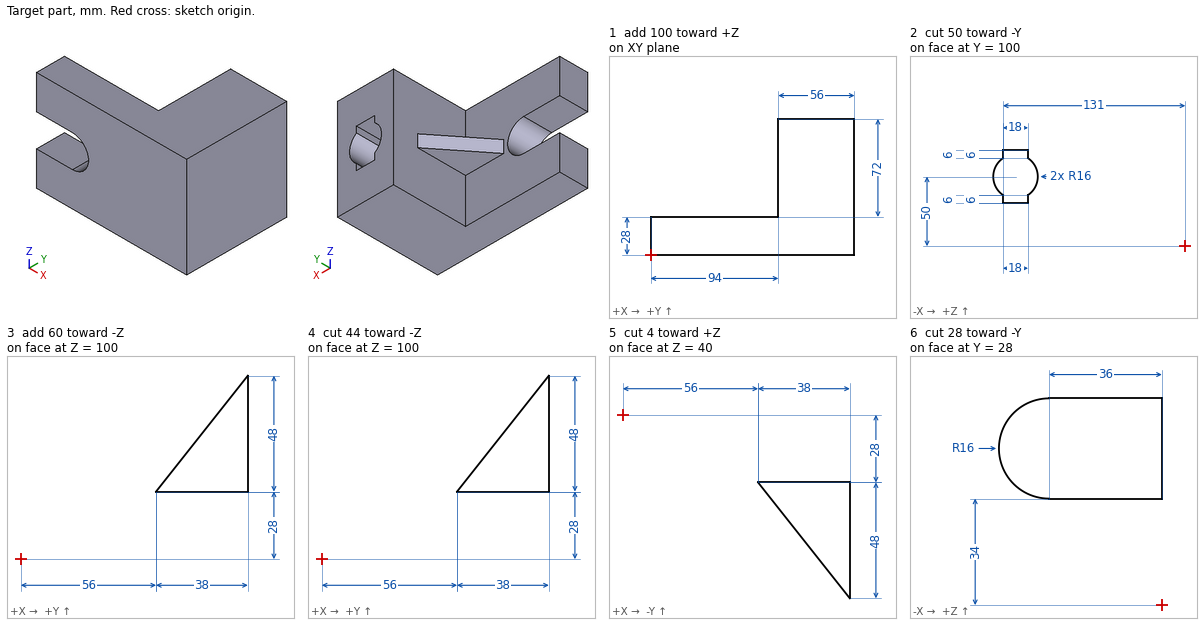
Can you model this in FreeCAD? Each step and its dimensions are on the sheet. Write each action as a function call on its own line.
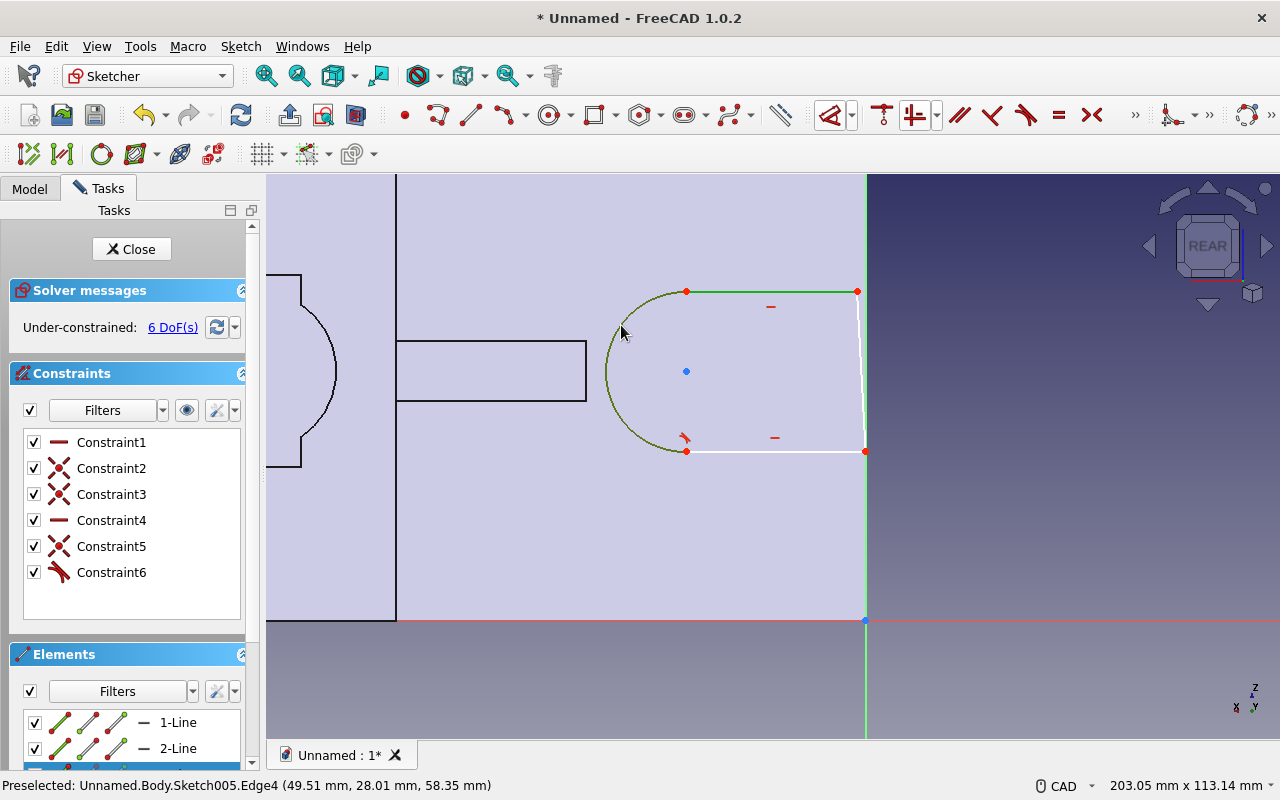
click(1026, 116)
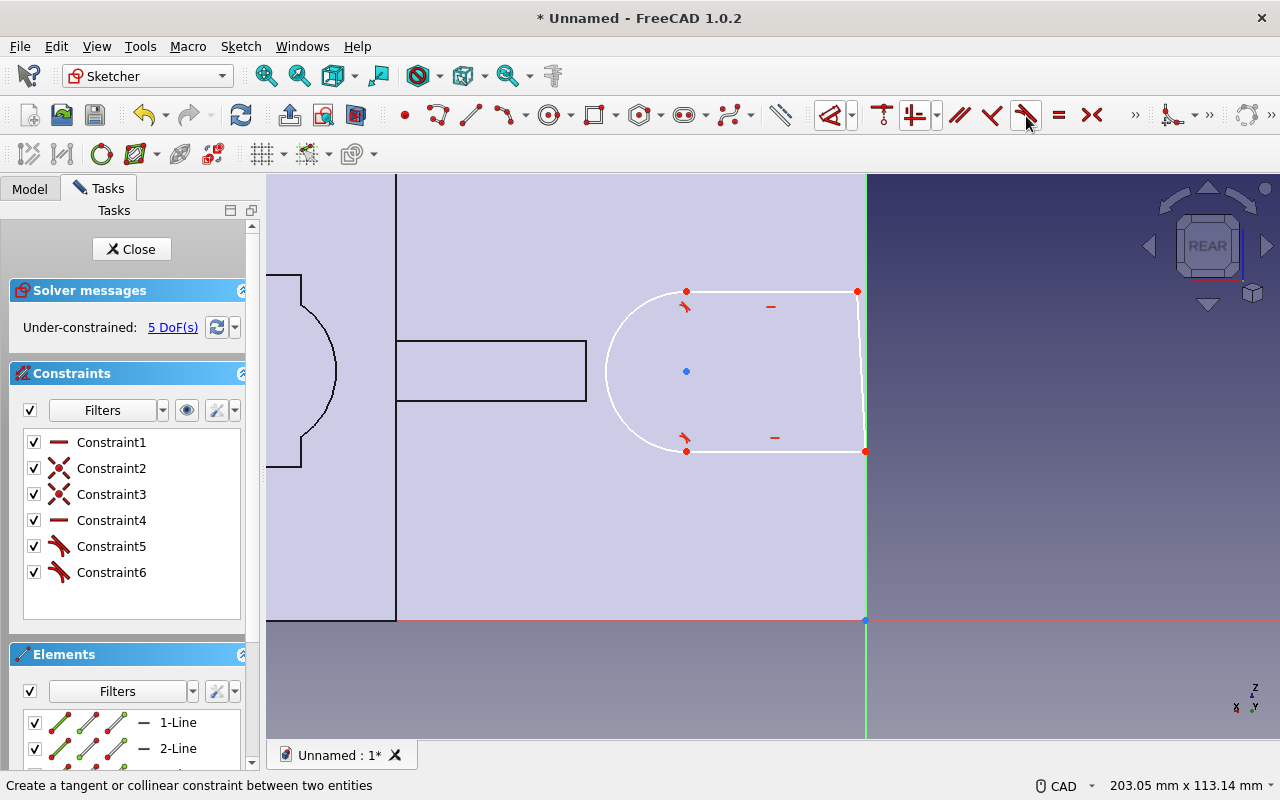
click(863, 404)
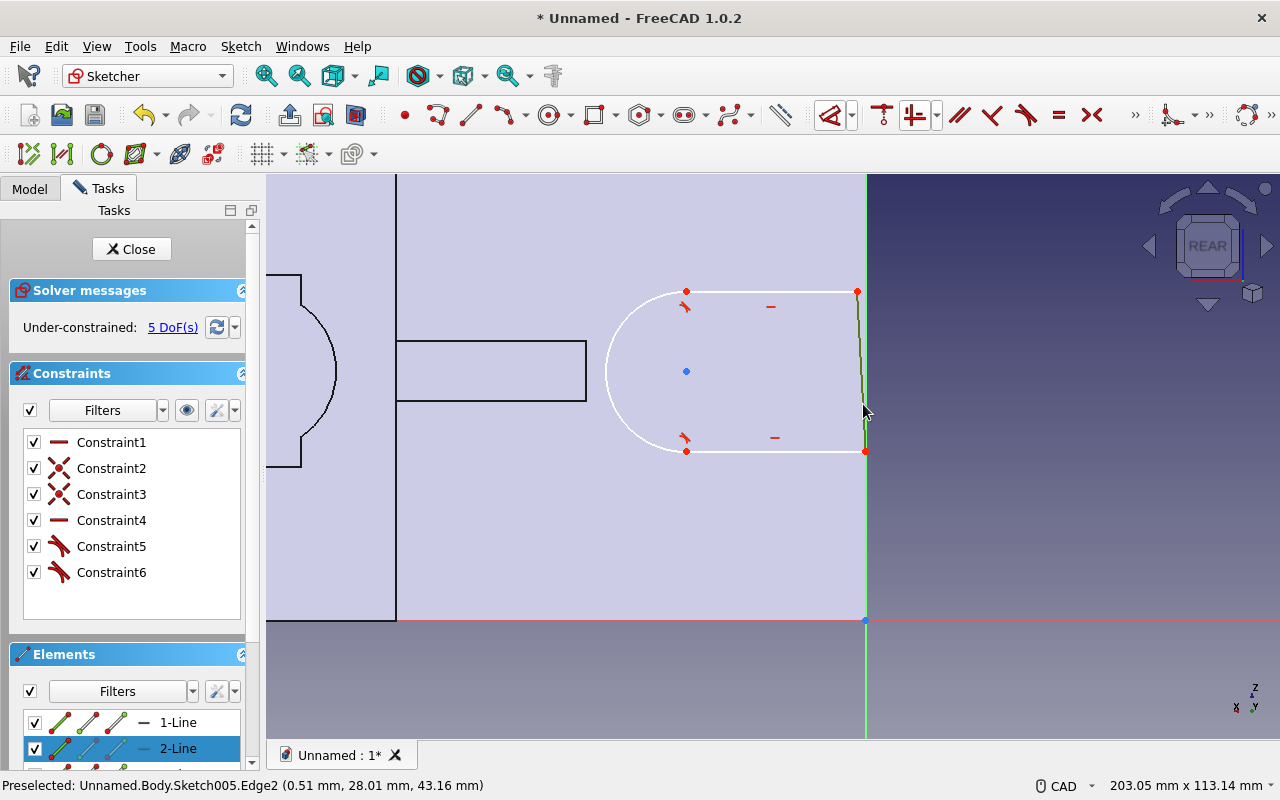
key(v)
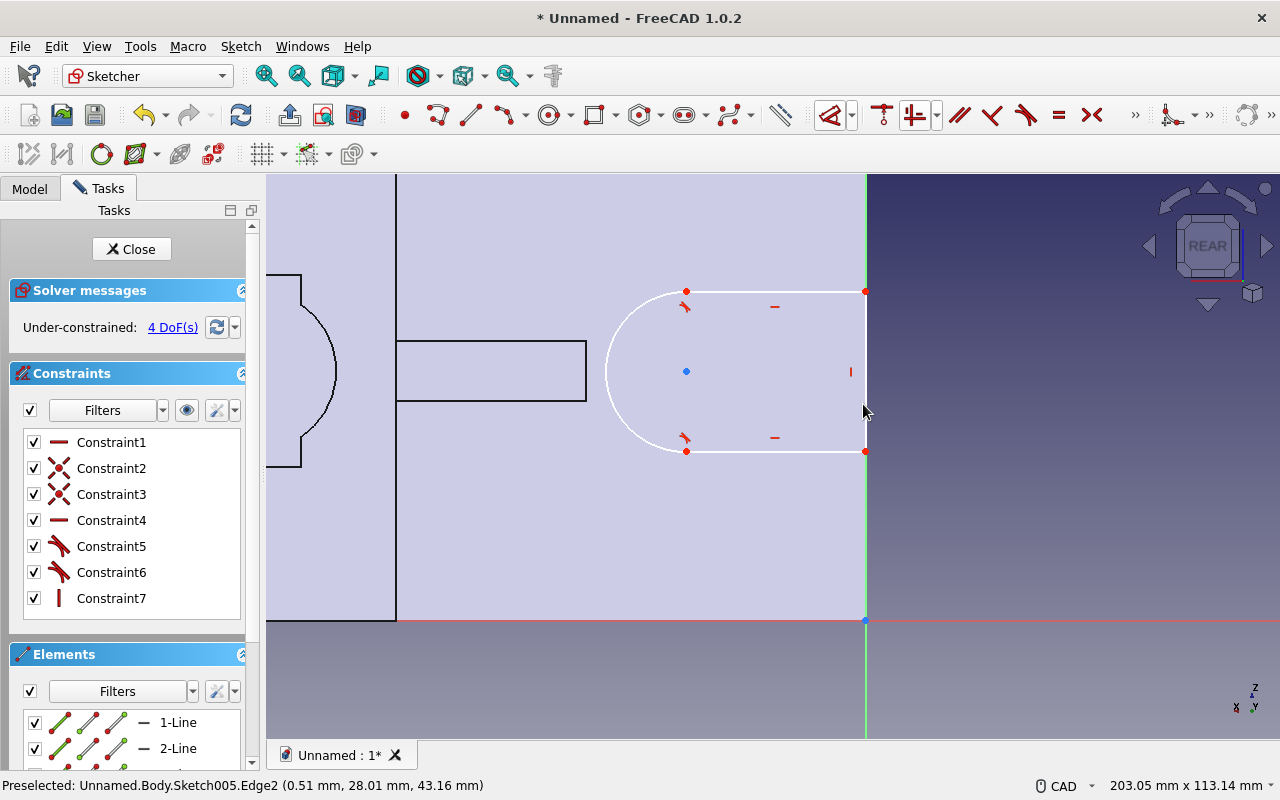
click(621, 325)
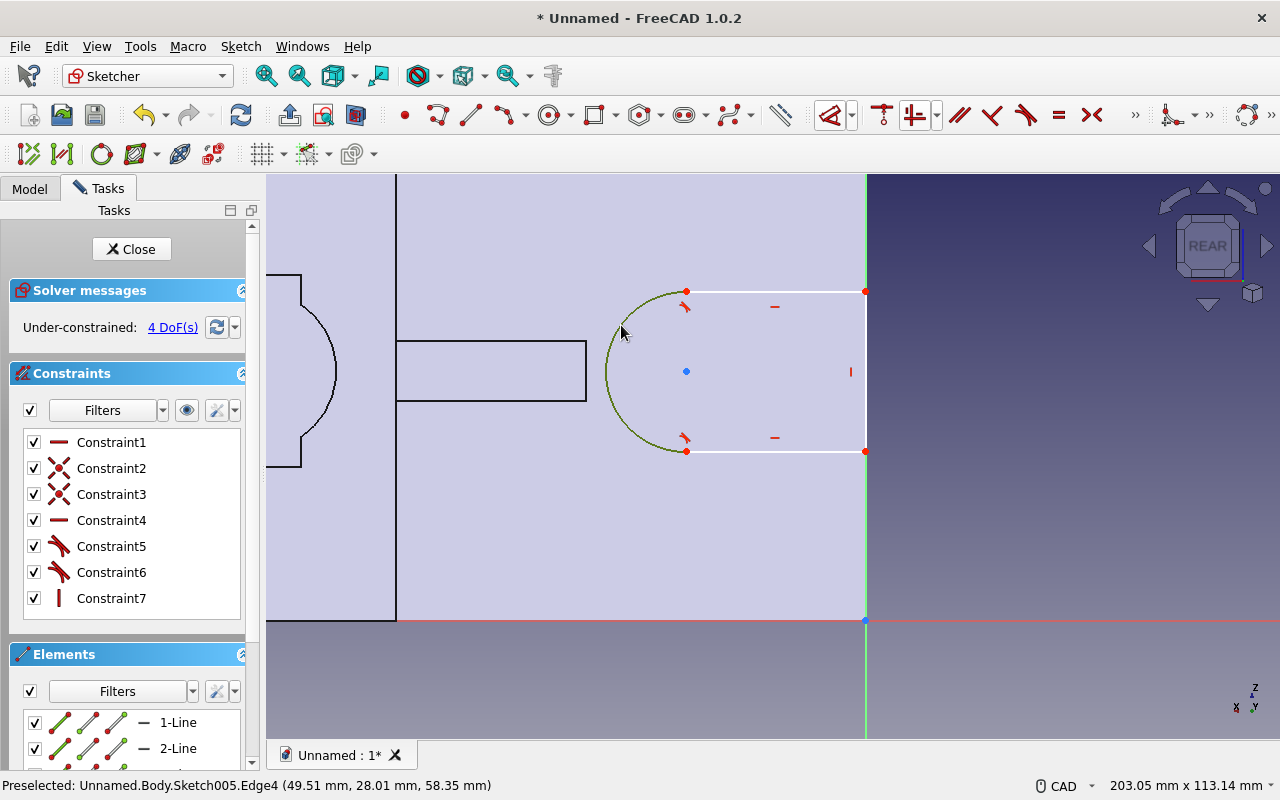
click(852, 116)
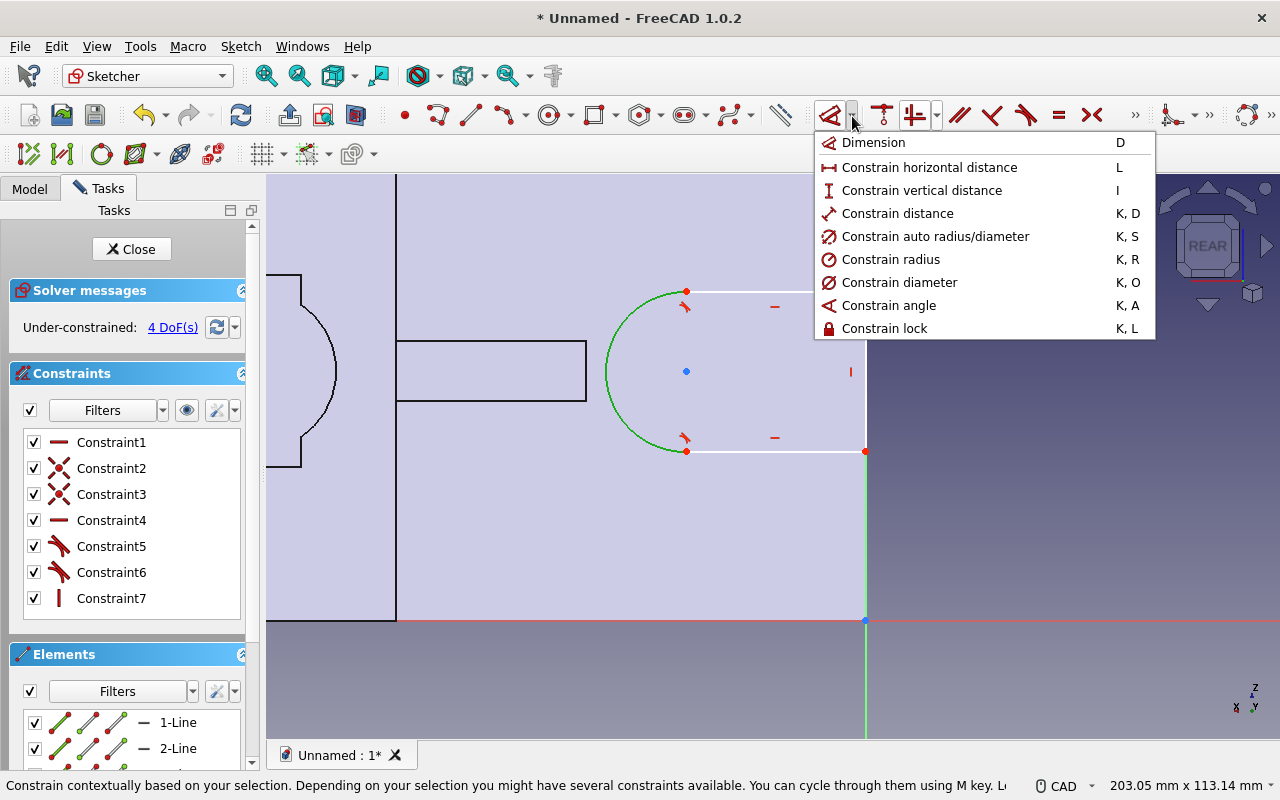
click(985, 260)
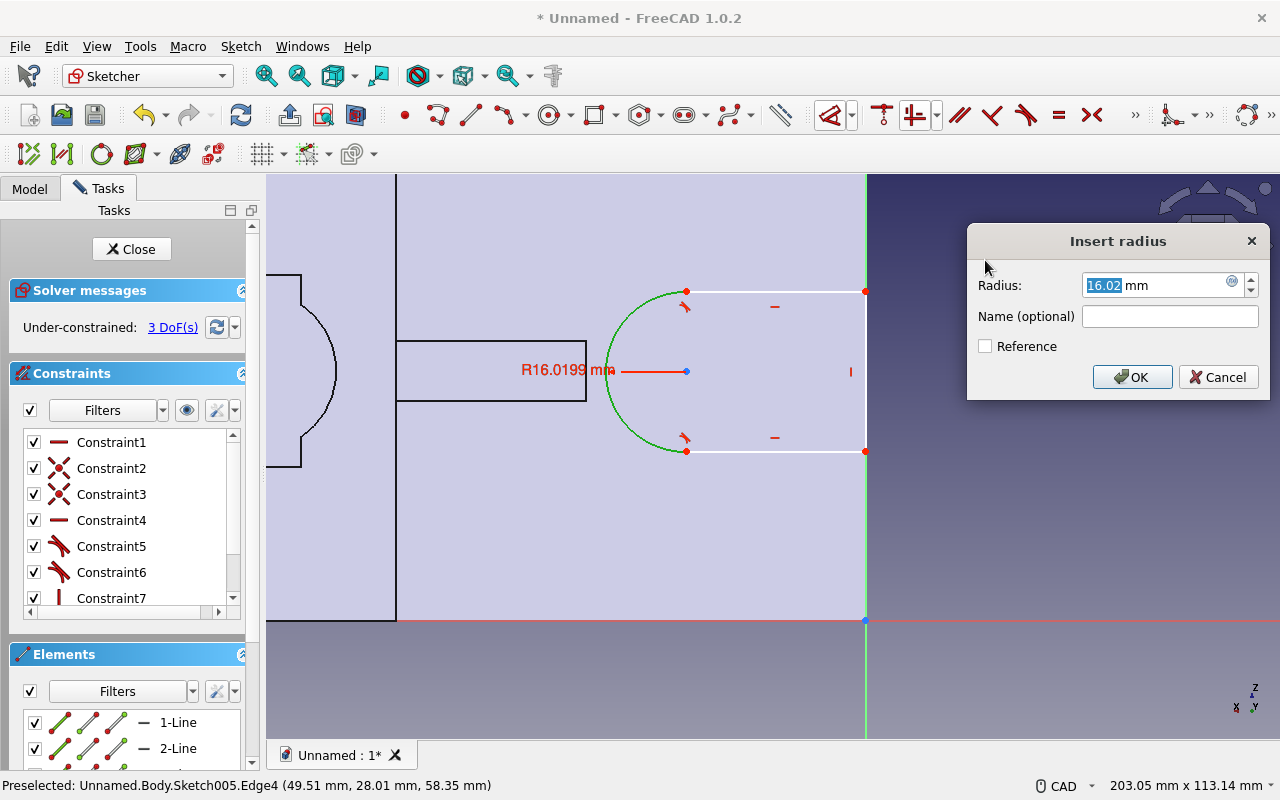
text(16)
key(Return)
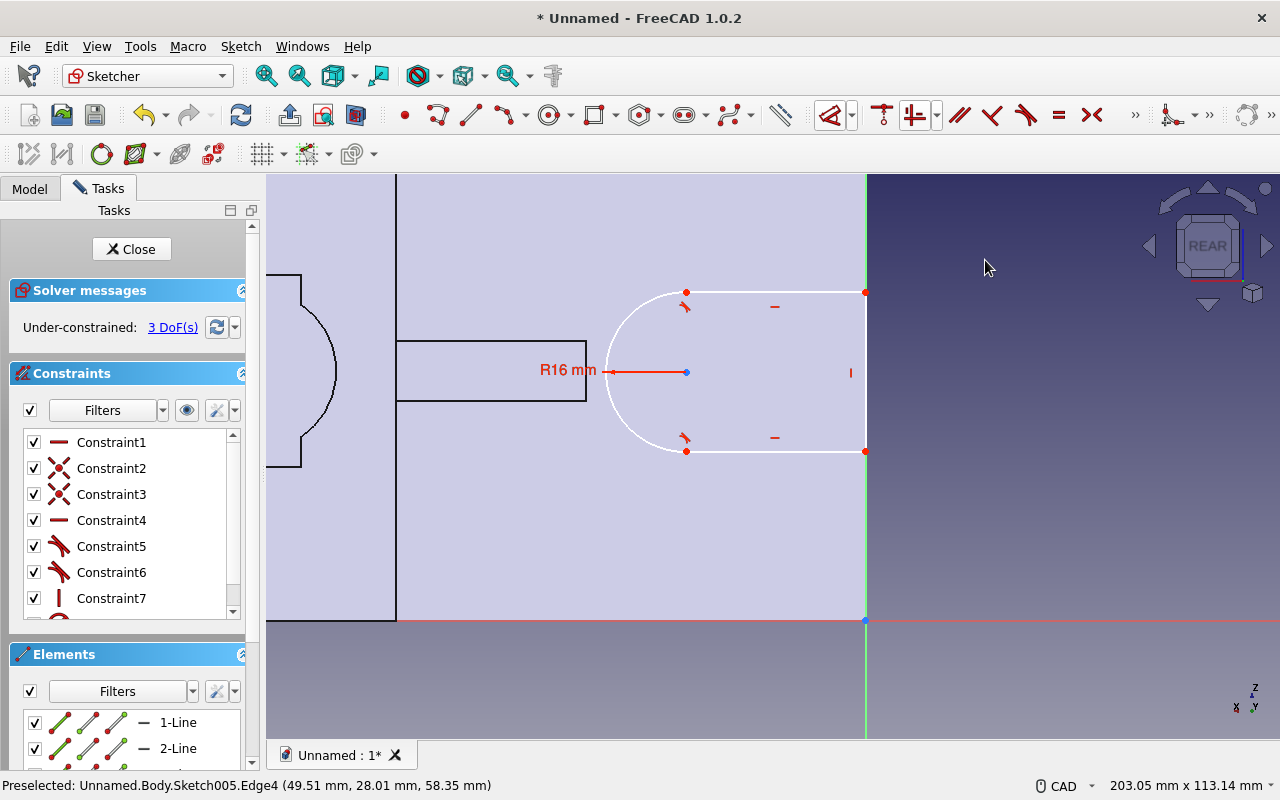
click(866, 452)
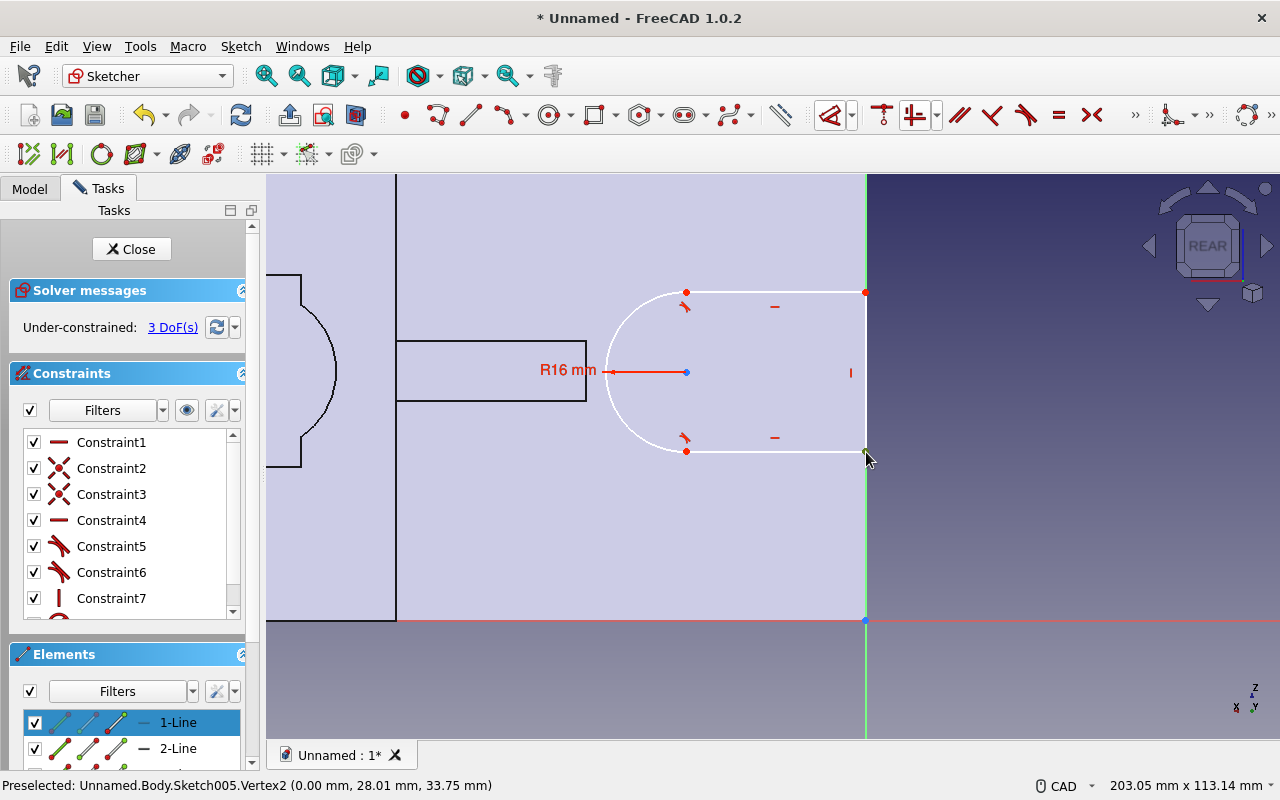
click(866, 675)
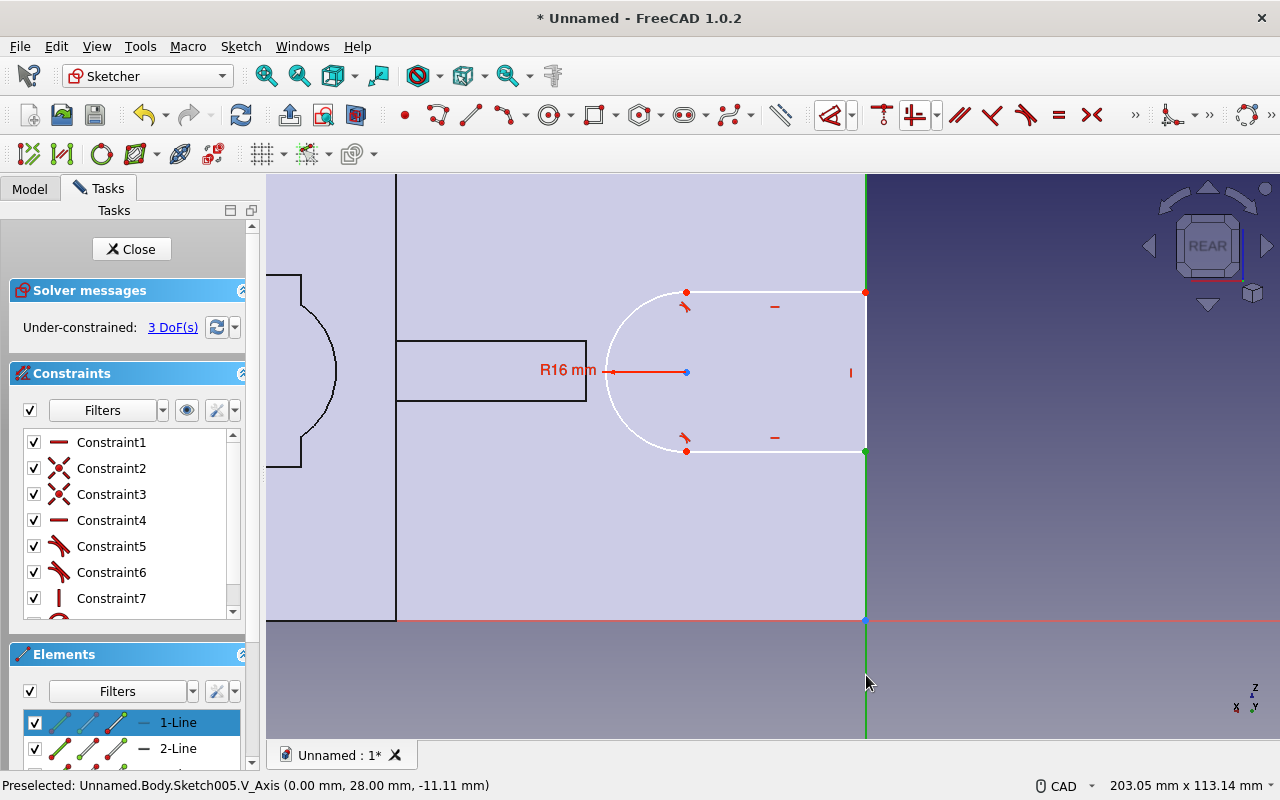
click(882, 116)